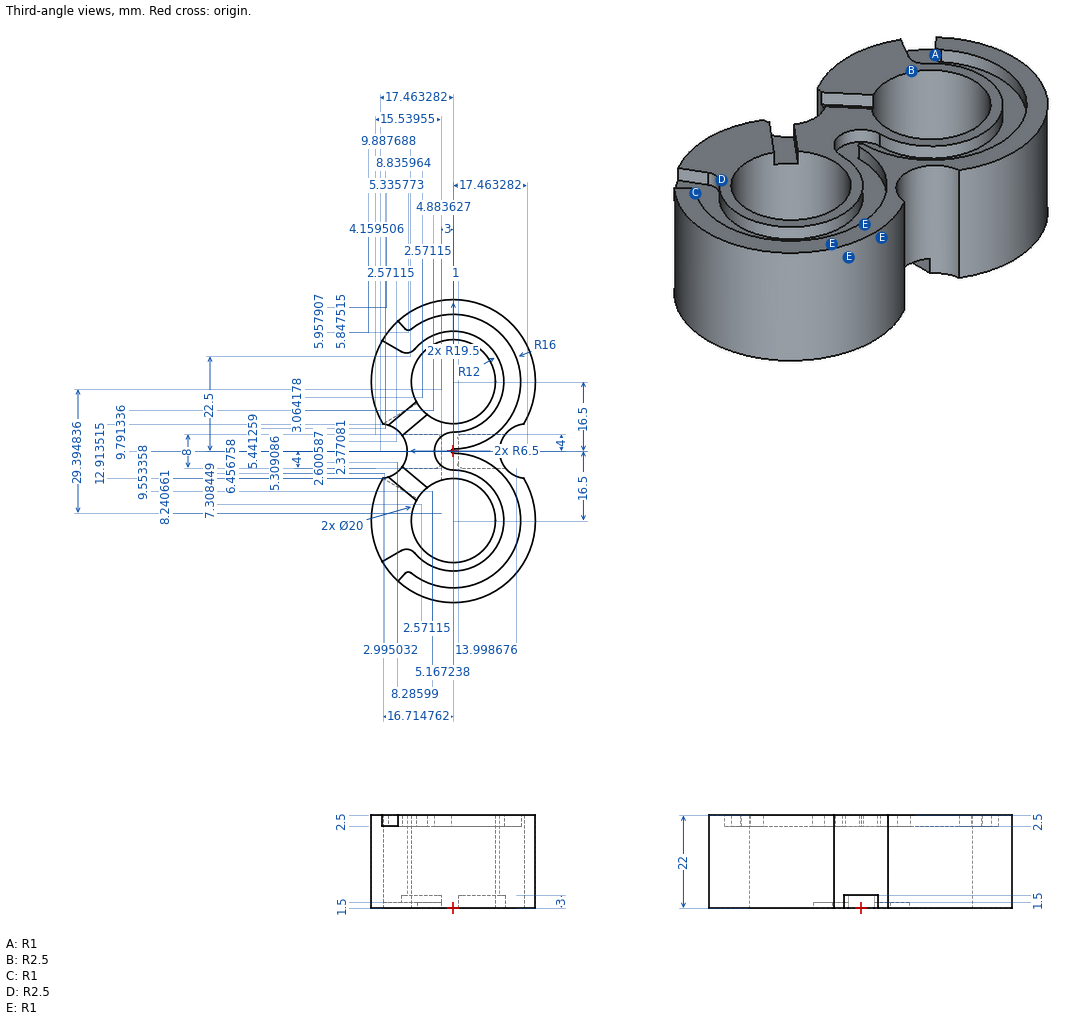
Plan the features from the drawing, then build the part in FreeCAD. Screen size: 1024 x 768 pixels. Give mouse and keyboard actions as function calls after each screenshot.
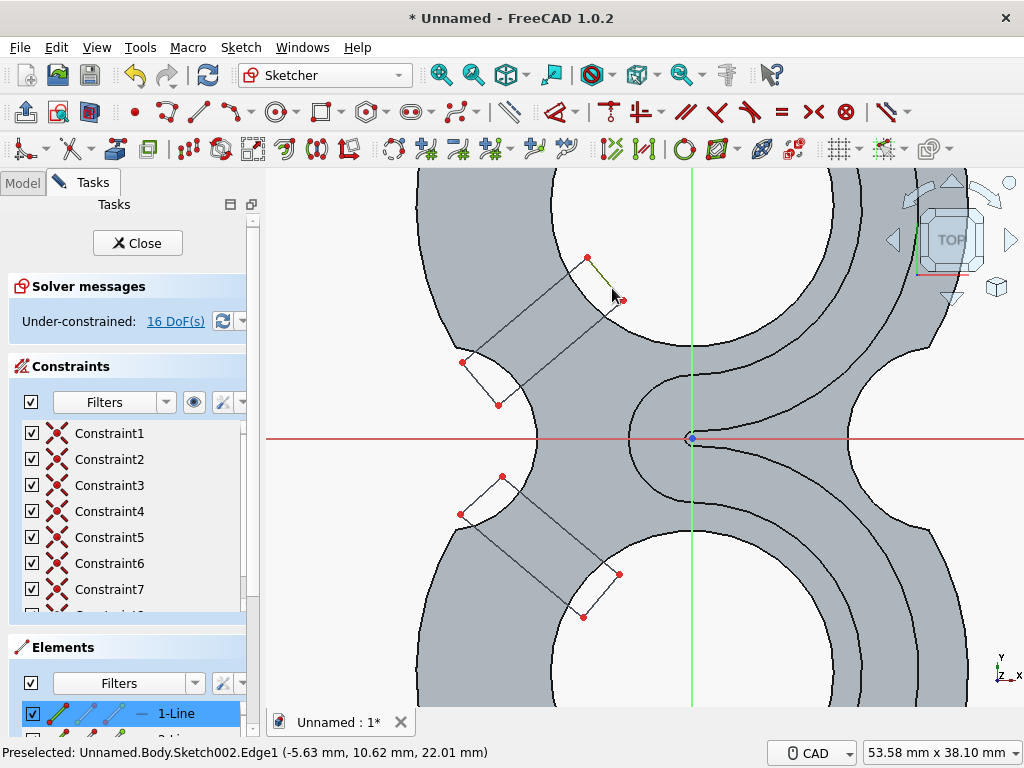
click(578, 112)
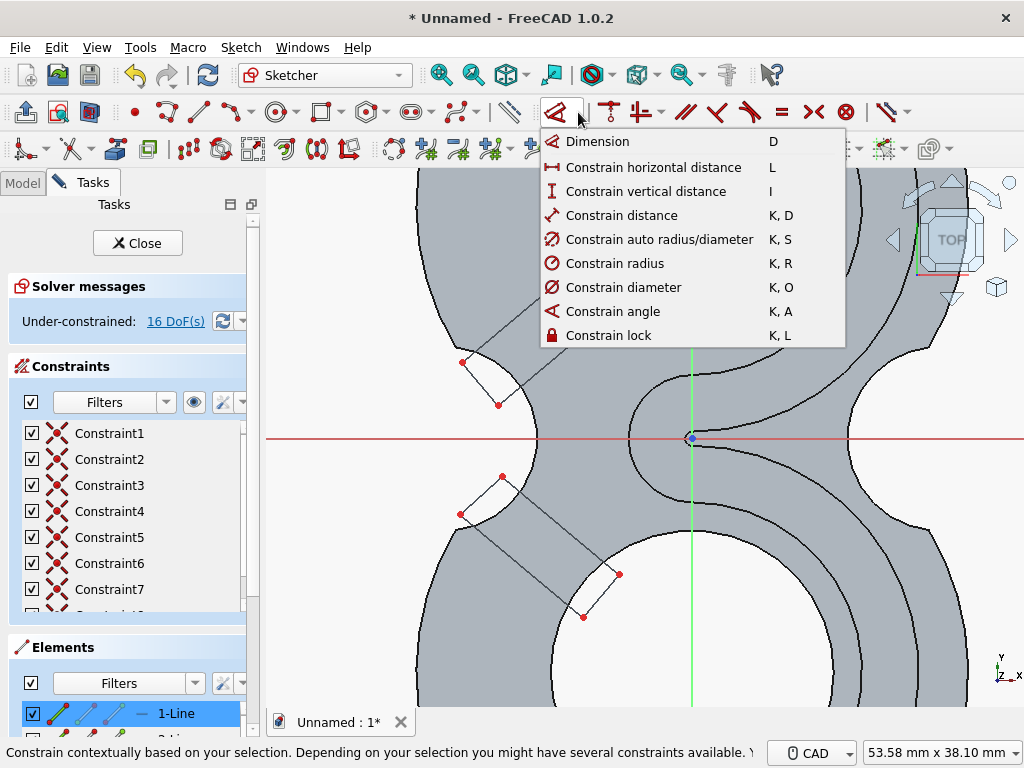
click(693, 167)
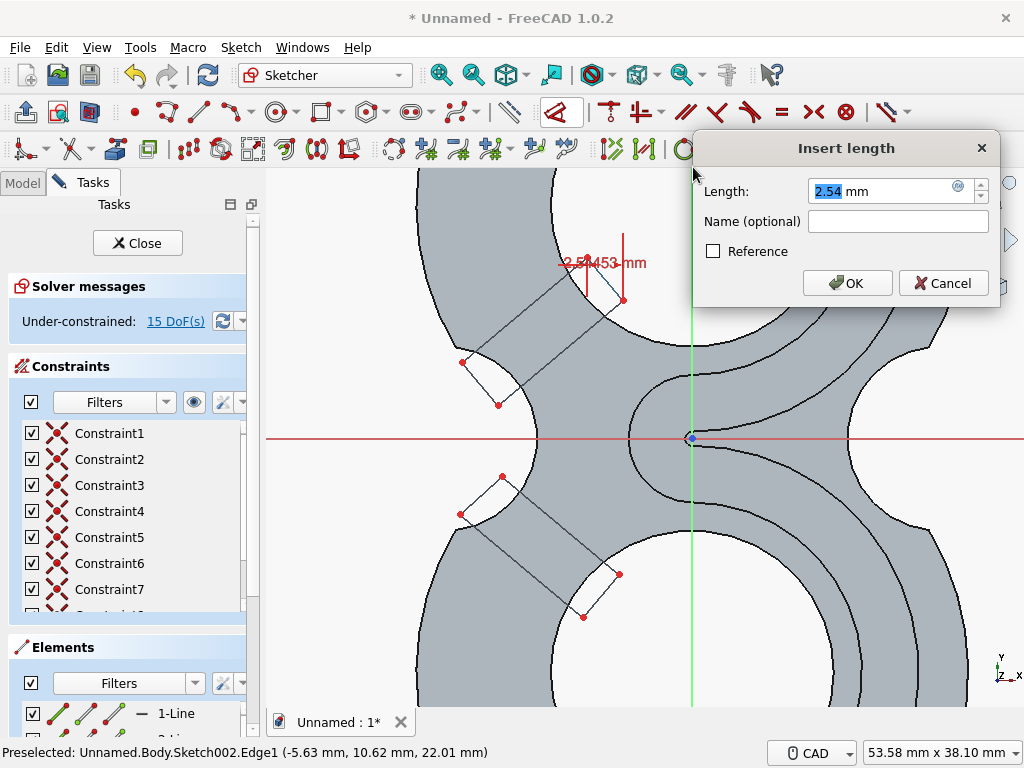
text(2.57115)
key(Return)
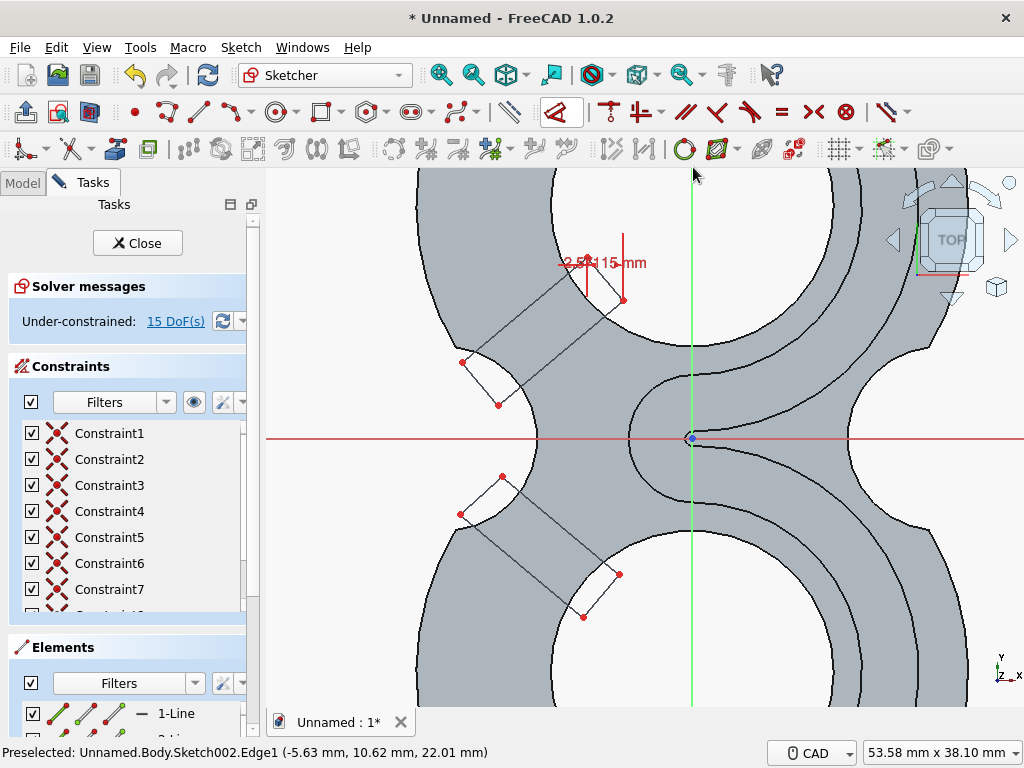
click(473, 376)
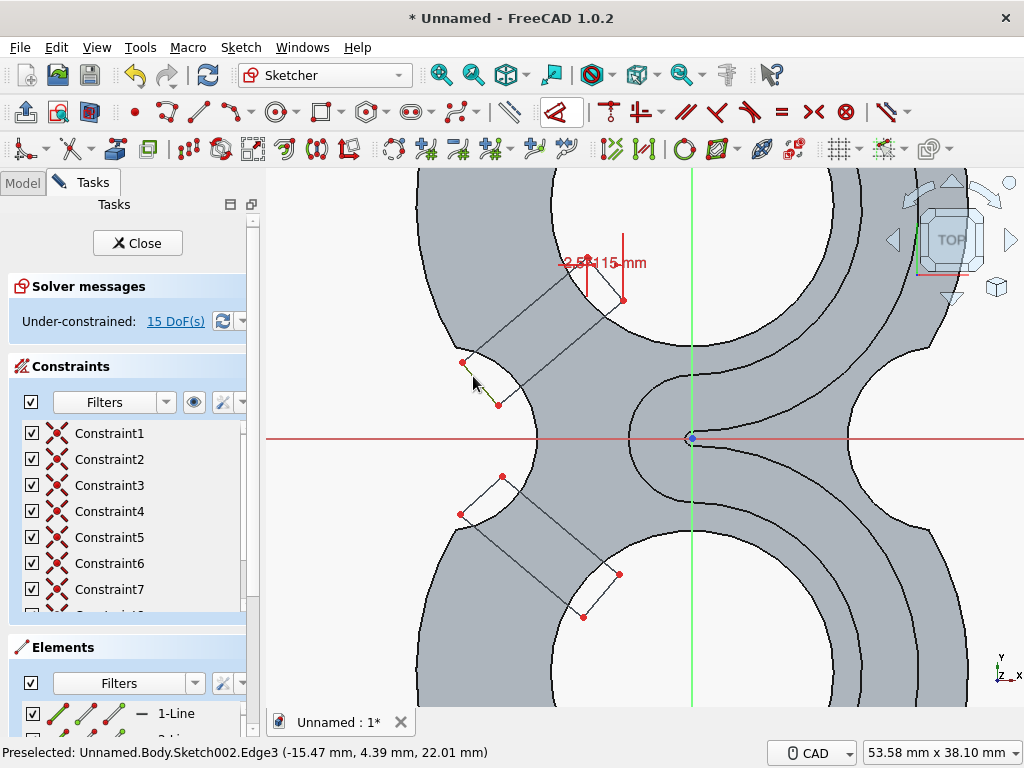
key(l)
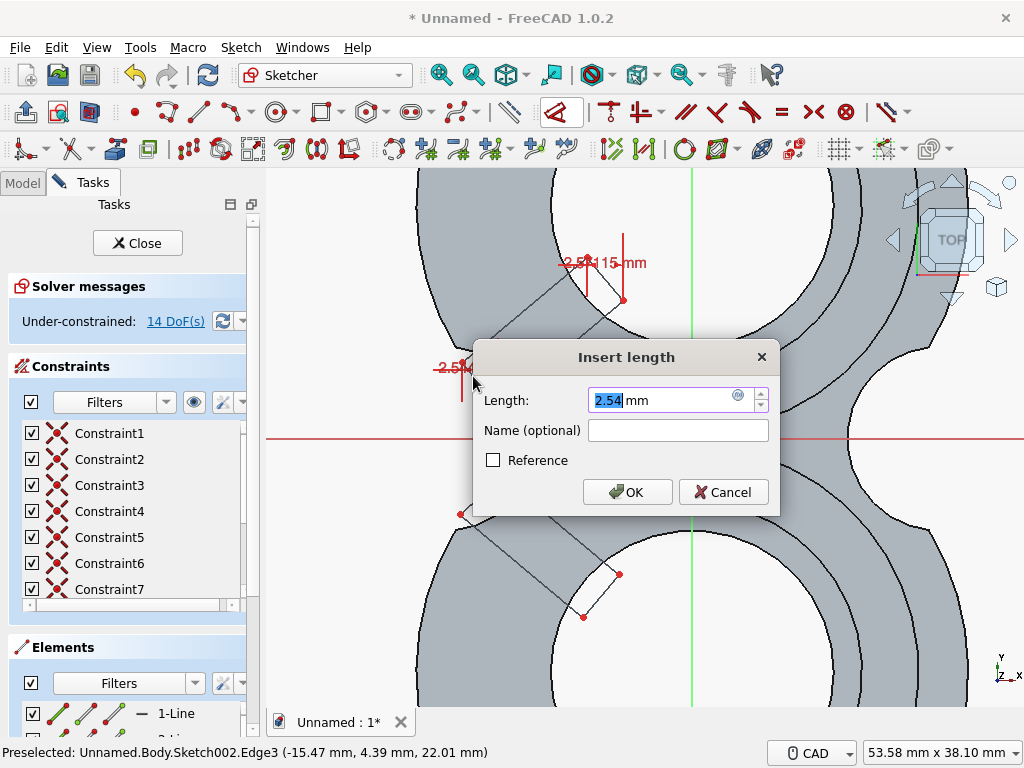
text(2.57115)
key(Return)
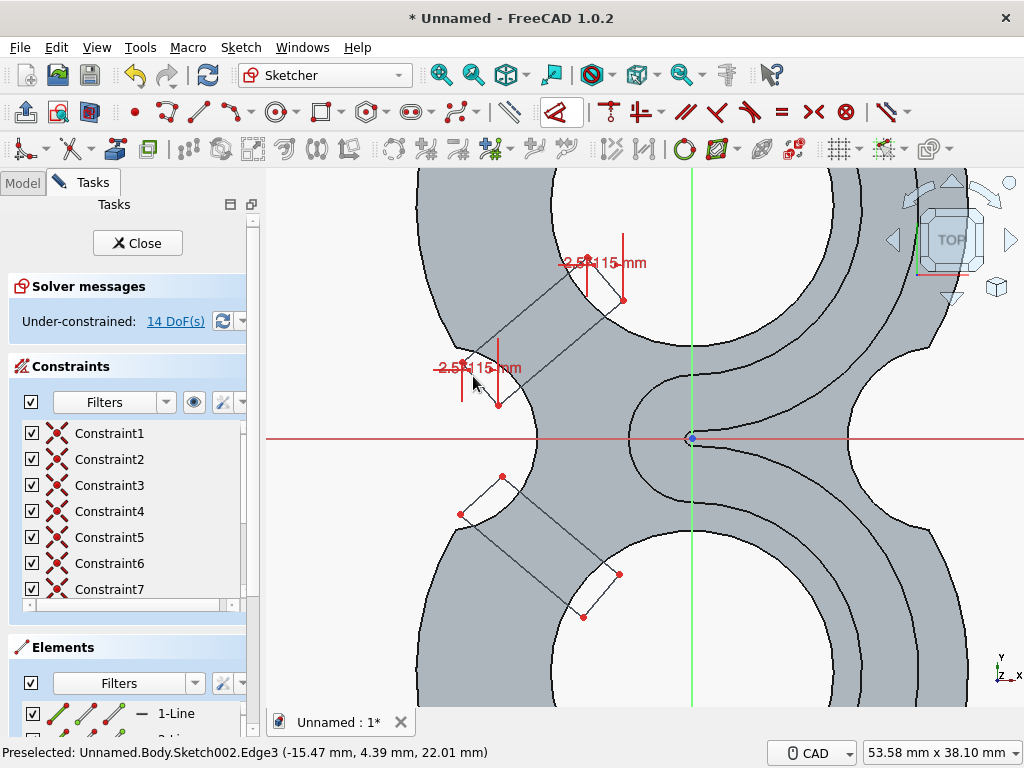
click(584, 546)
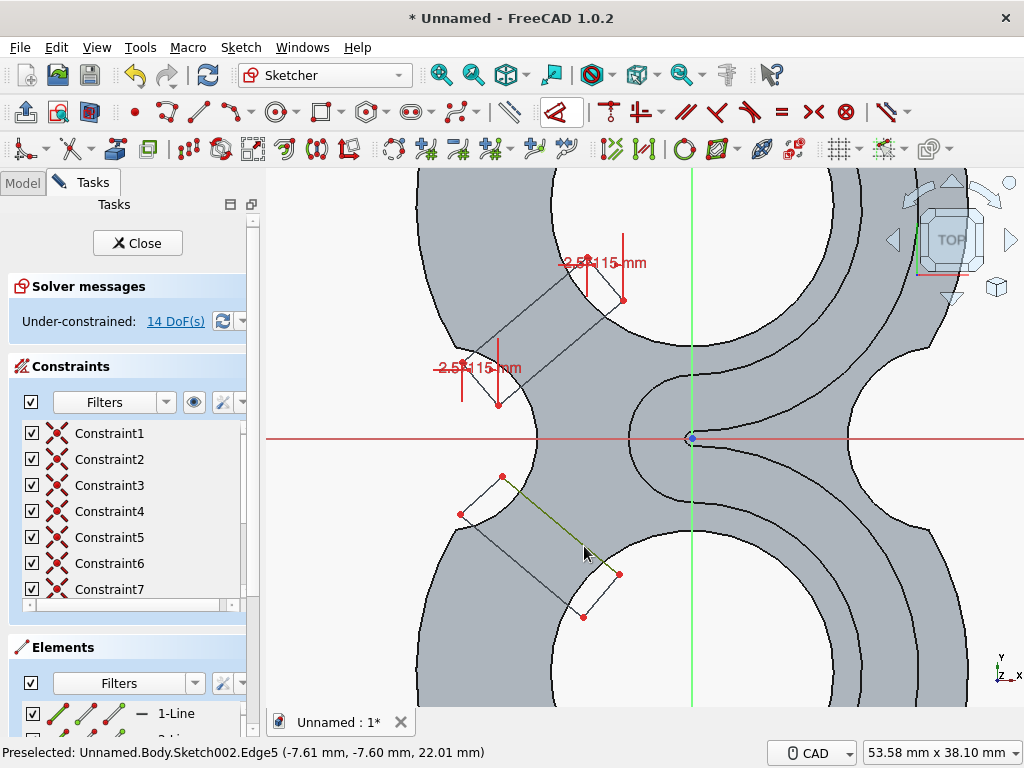
key(l)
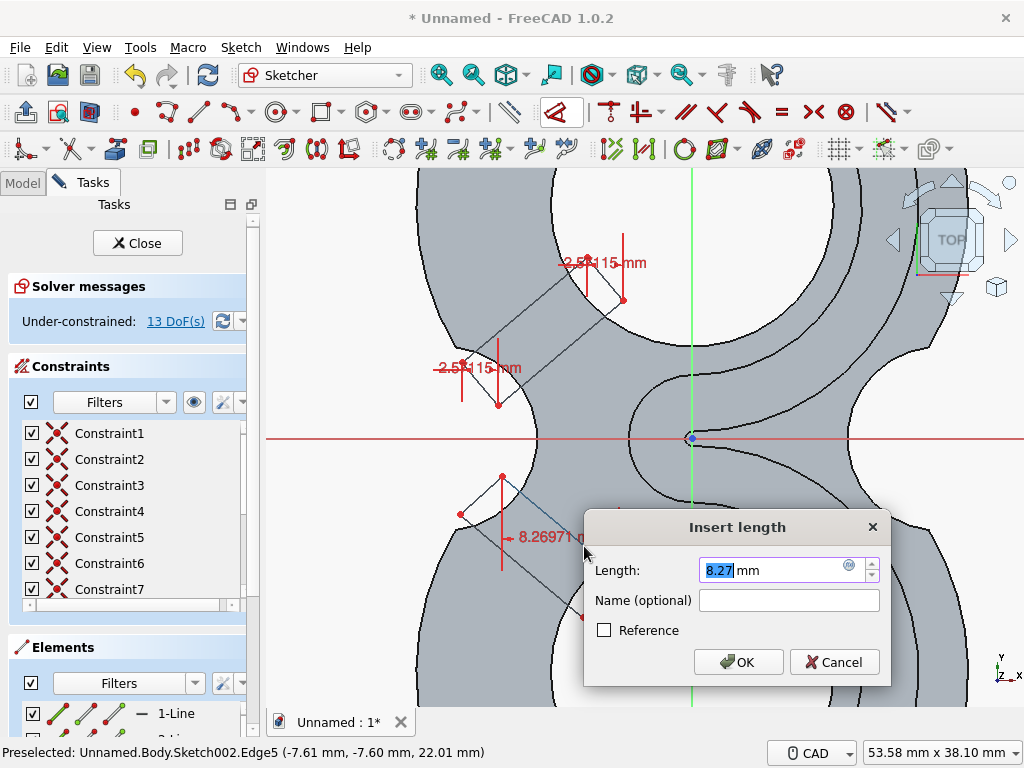
text(8.28599)
key(Return)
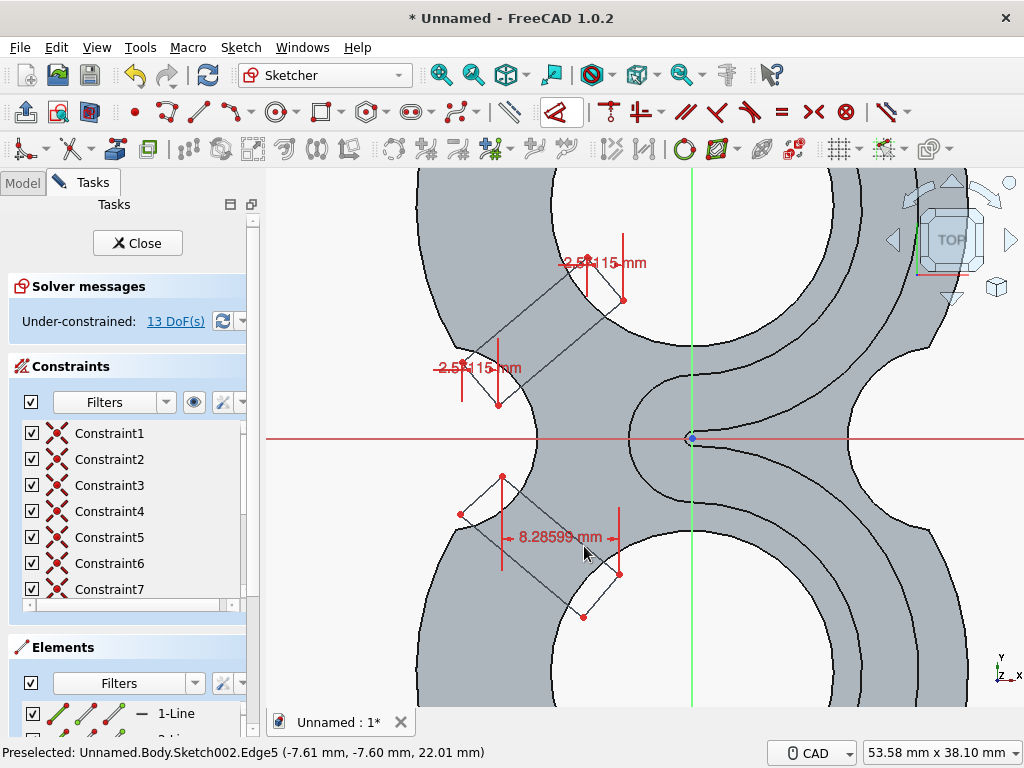
click(594, 605)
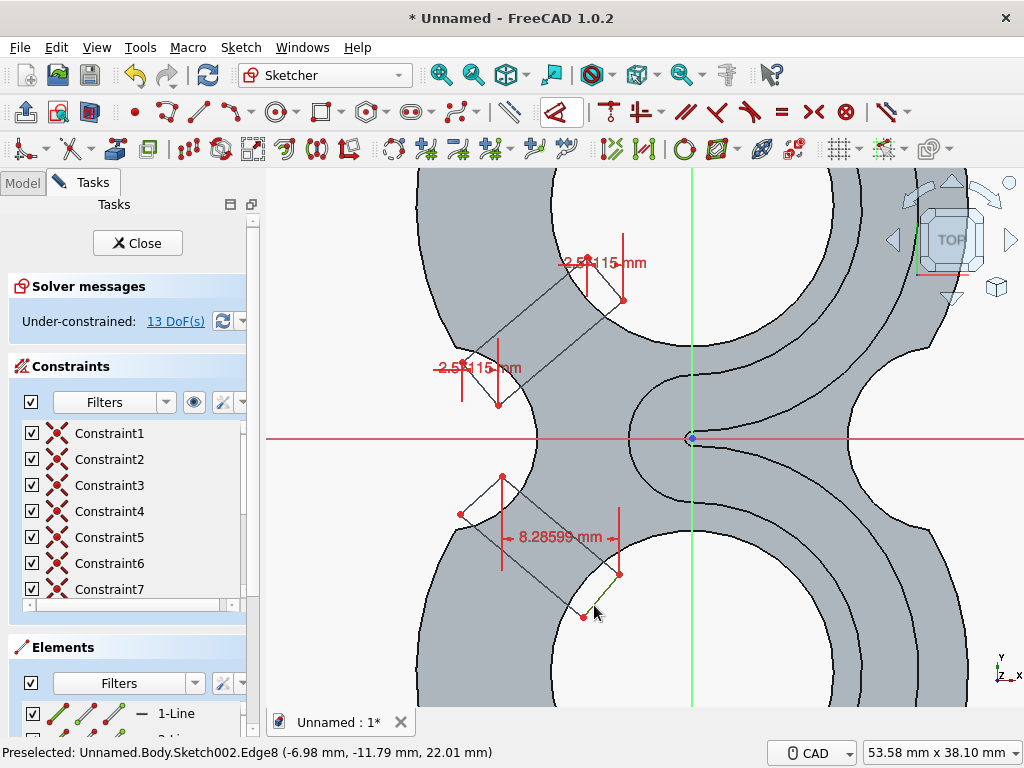
key(l)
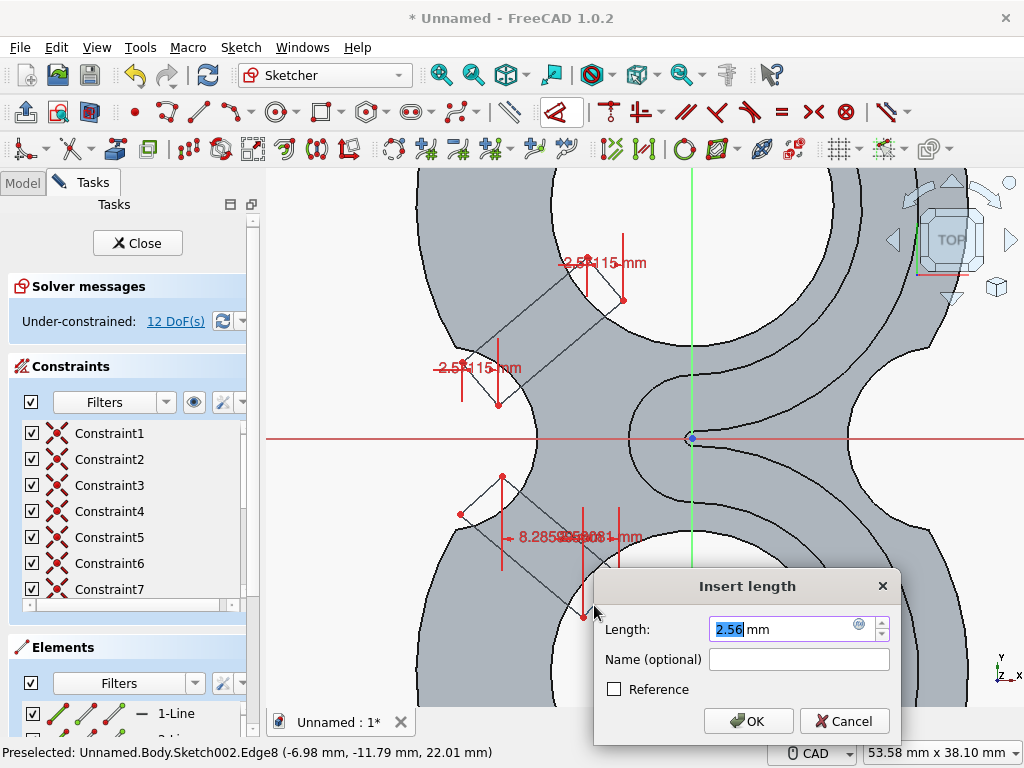
text(2.57115)
key(Return)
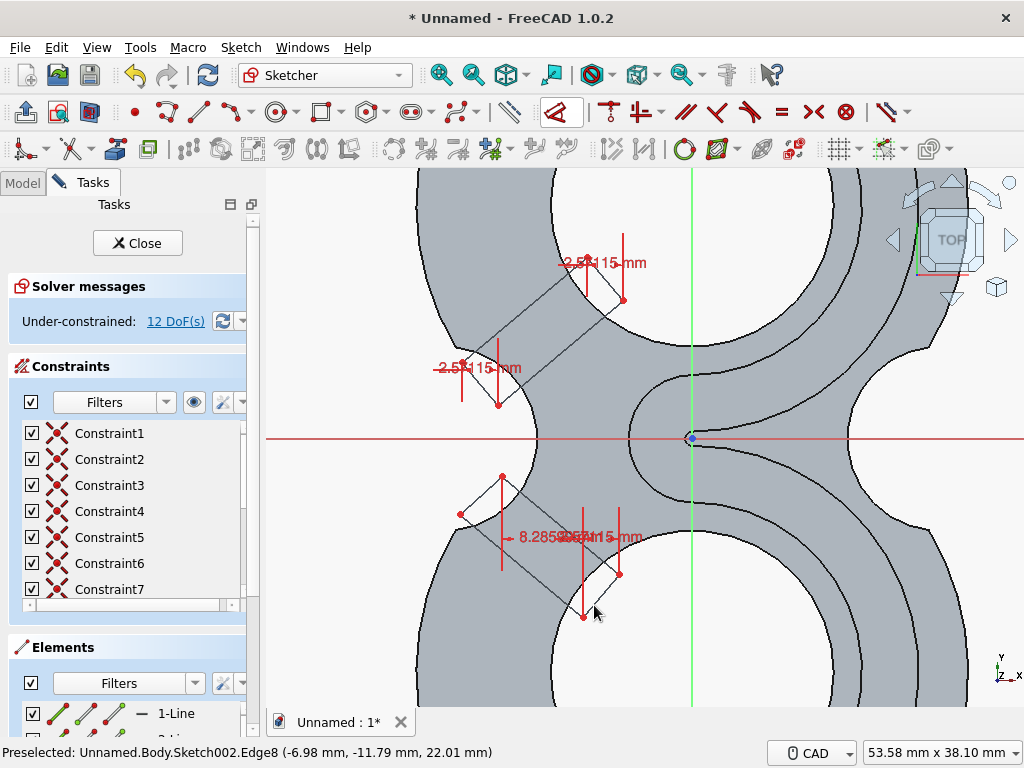
click(623, 301)